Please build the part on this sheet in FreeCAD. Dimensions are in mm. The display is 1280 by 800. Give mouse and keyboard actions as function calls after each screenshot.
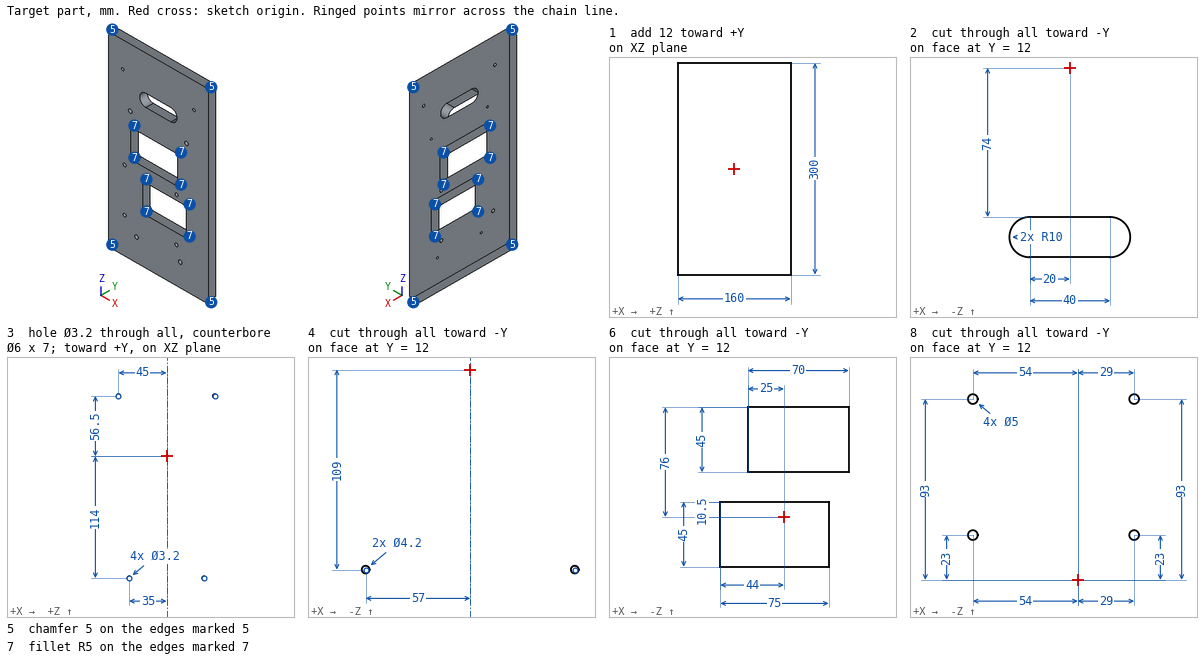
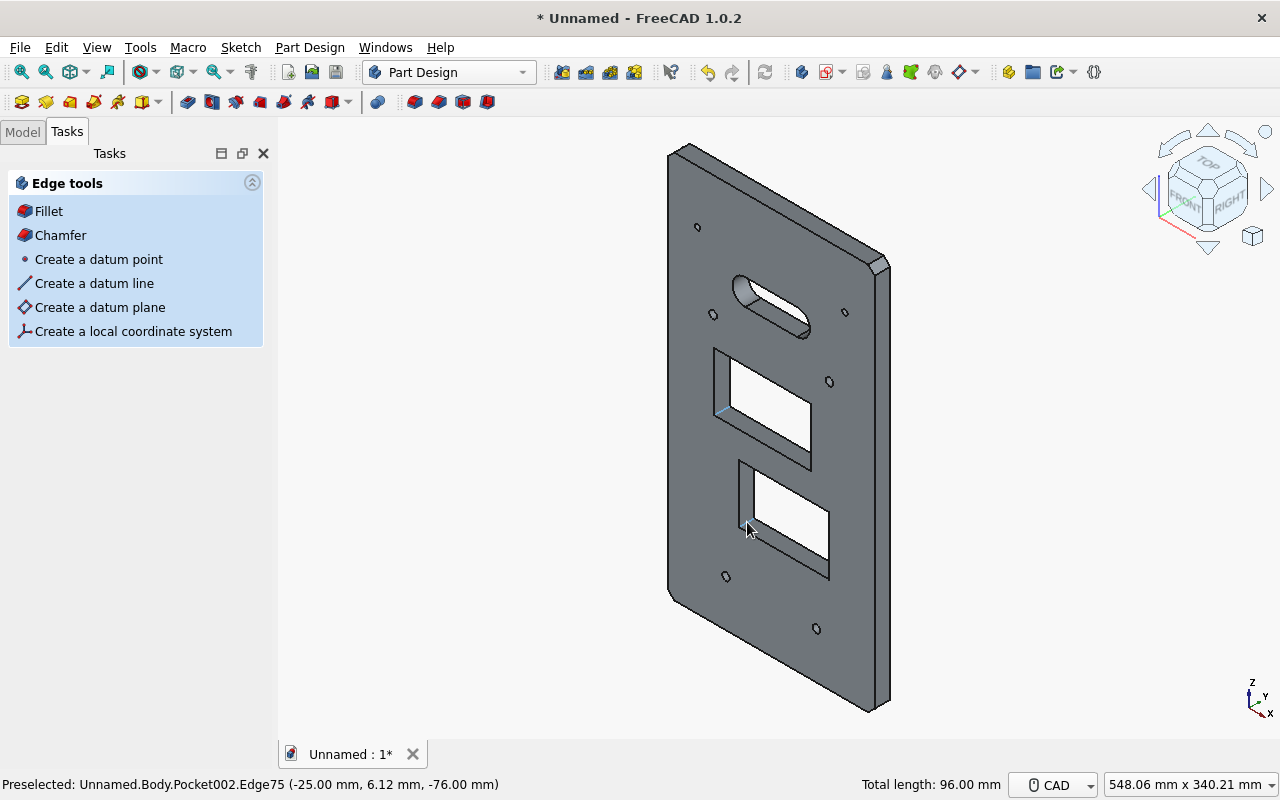
click(416, 102)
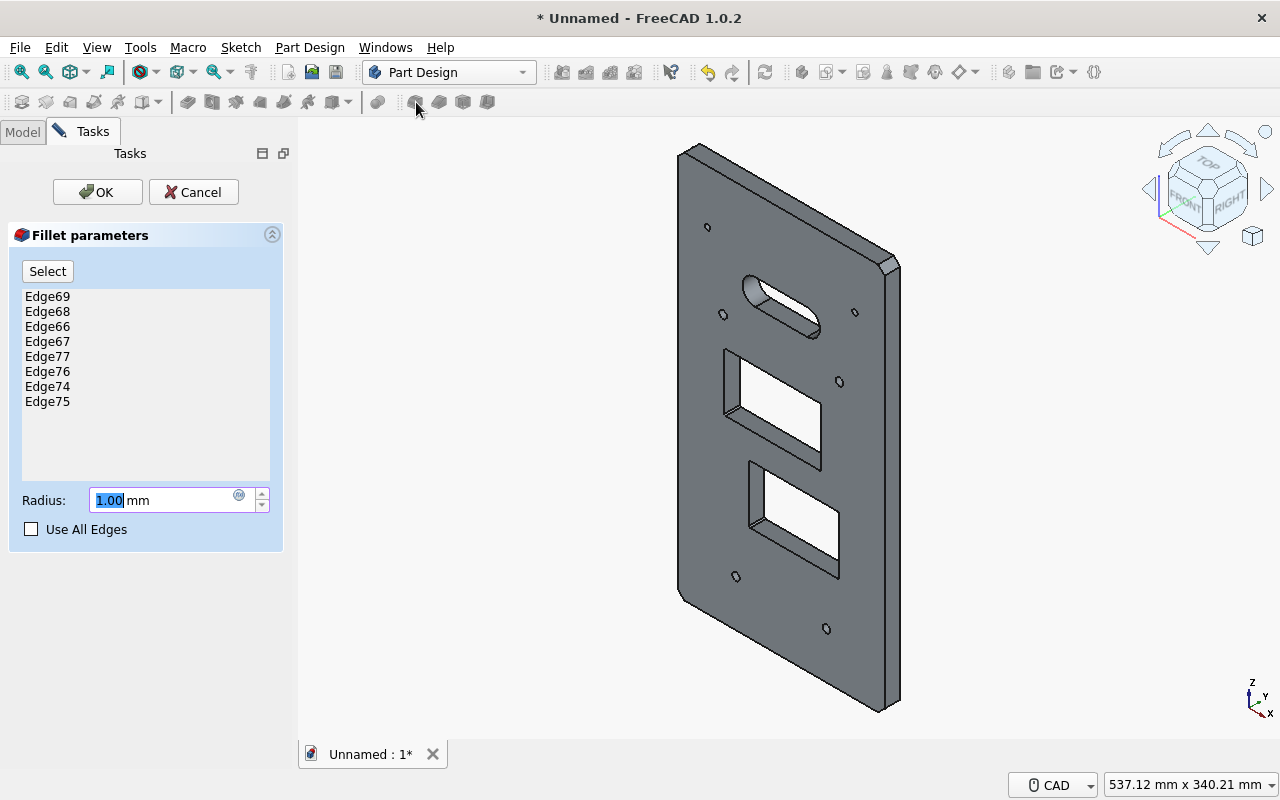
text(5)
key(Tab)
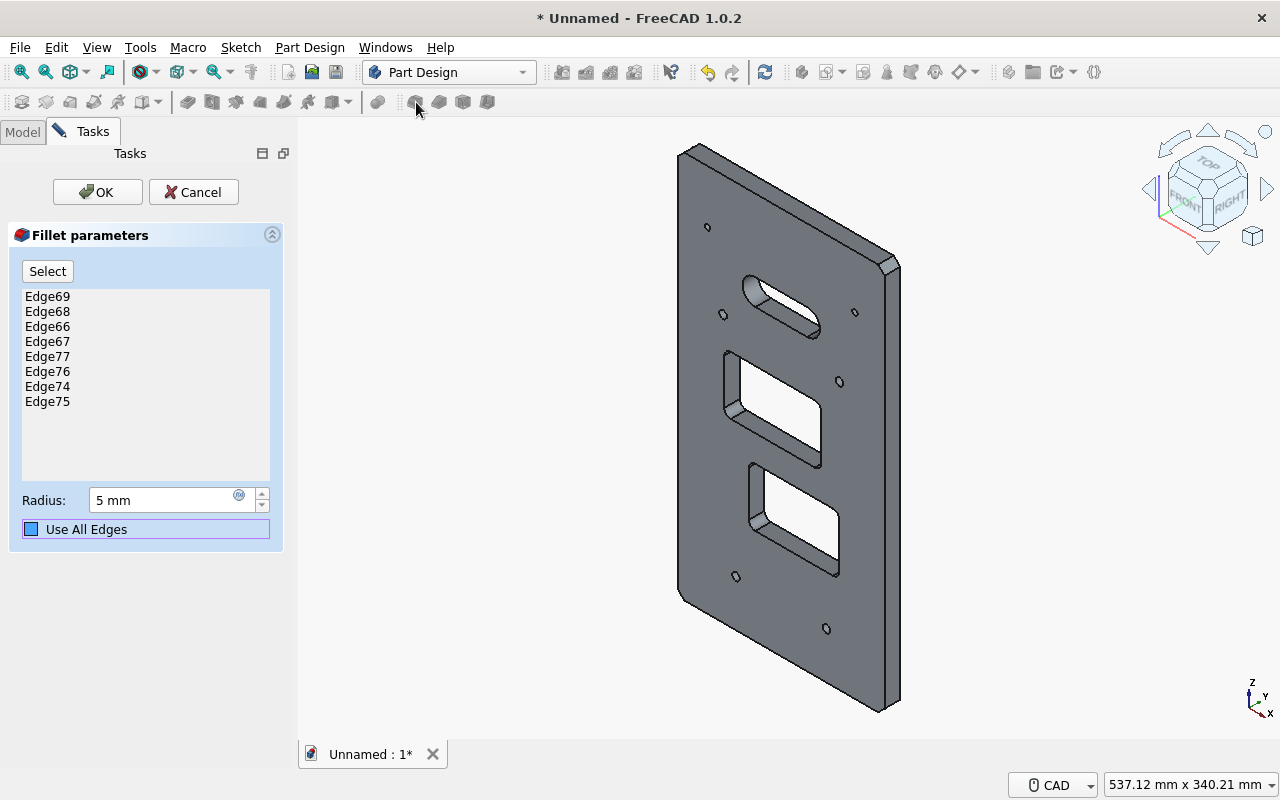
click(98, 192)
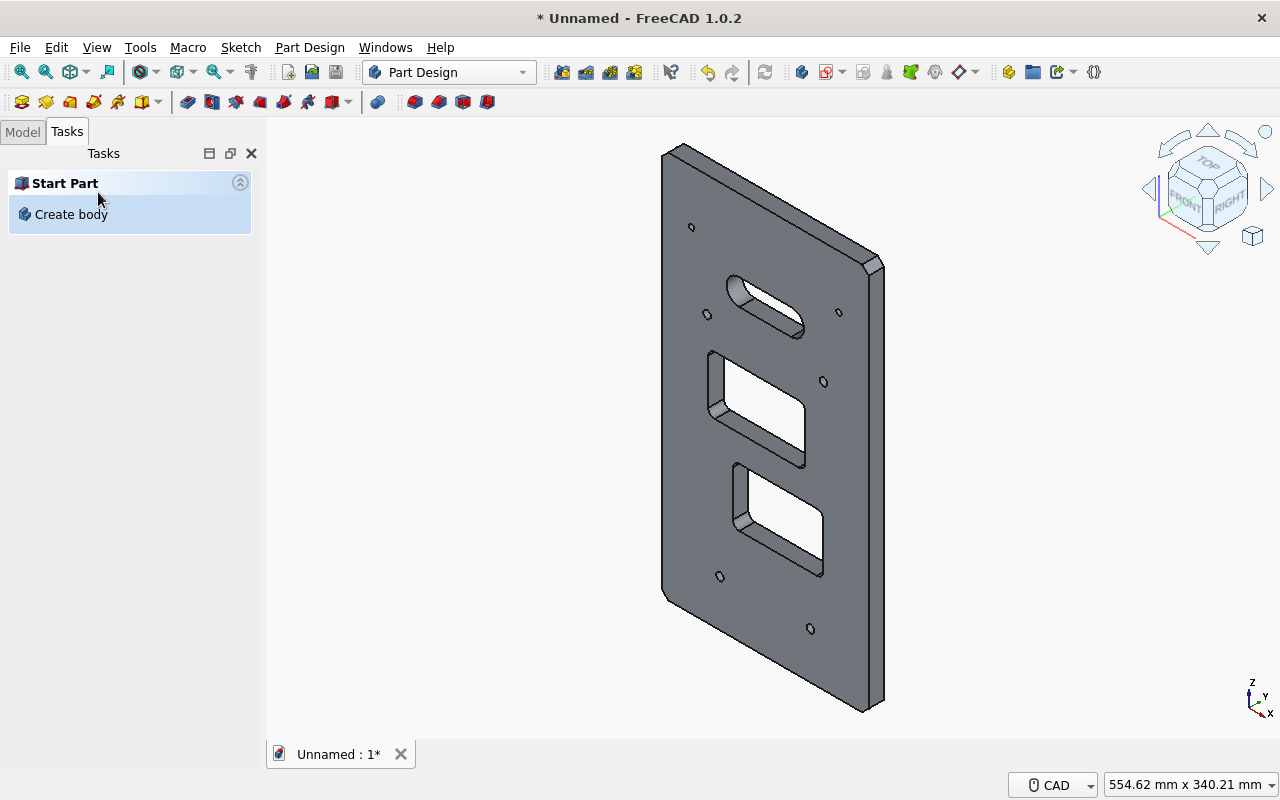
key(4)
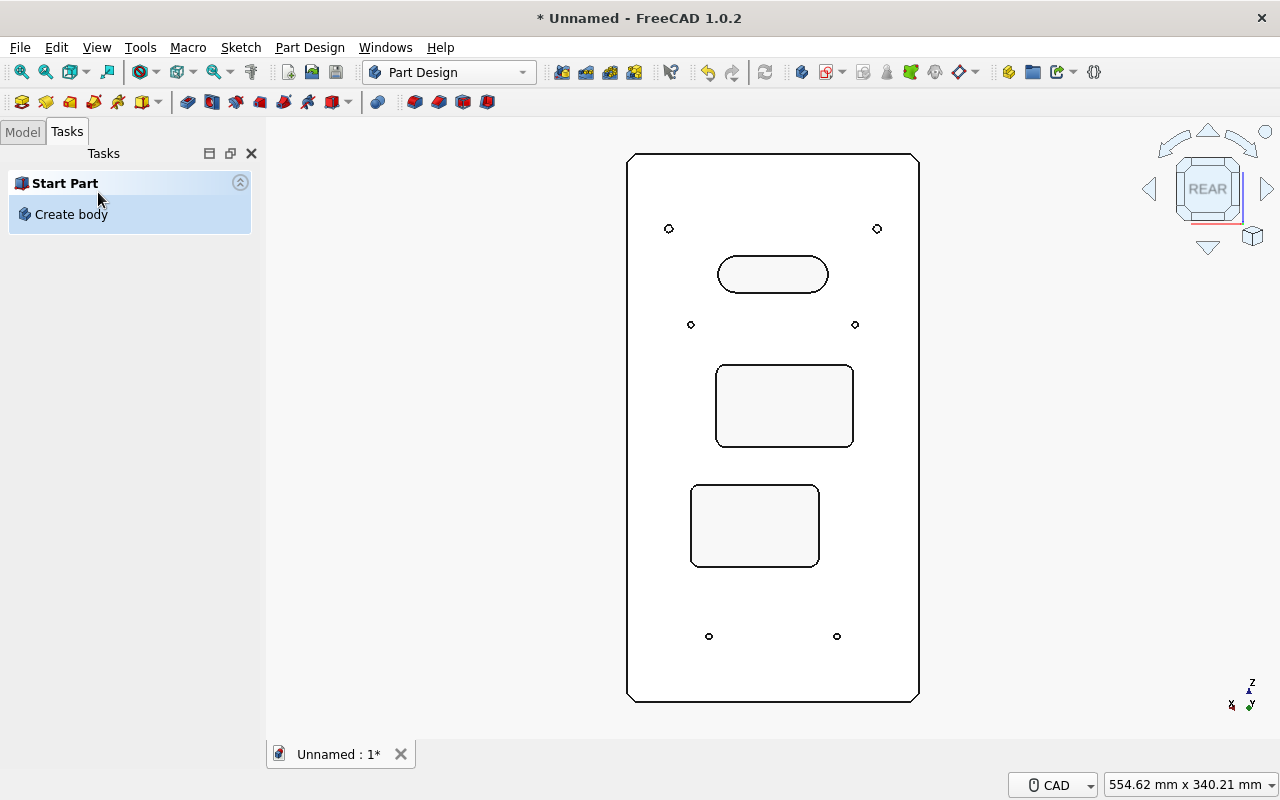
click(857, 584)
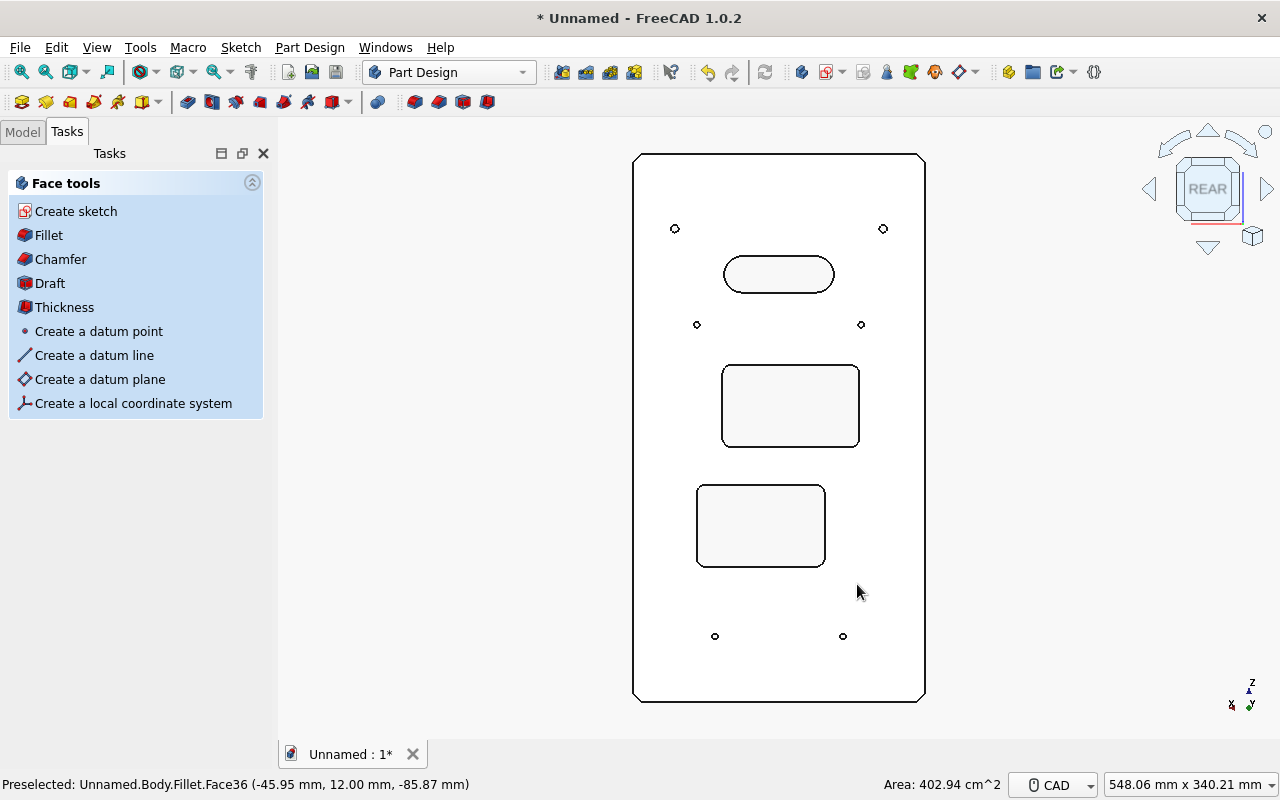
click(826, 72)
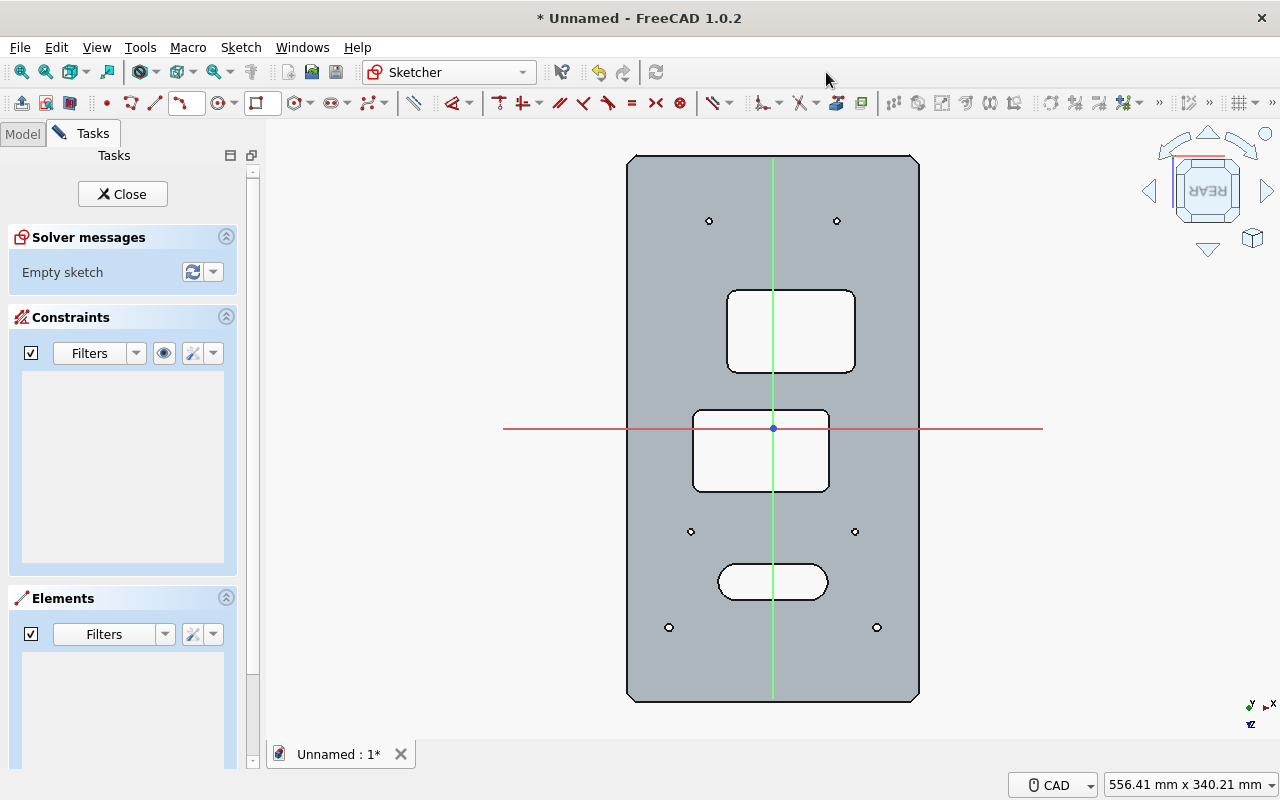
scroll(788, 271, up, 4)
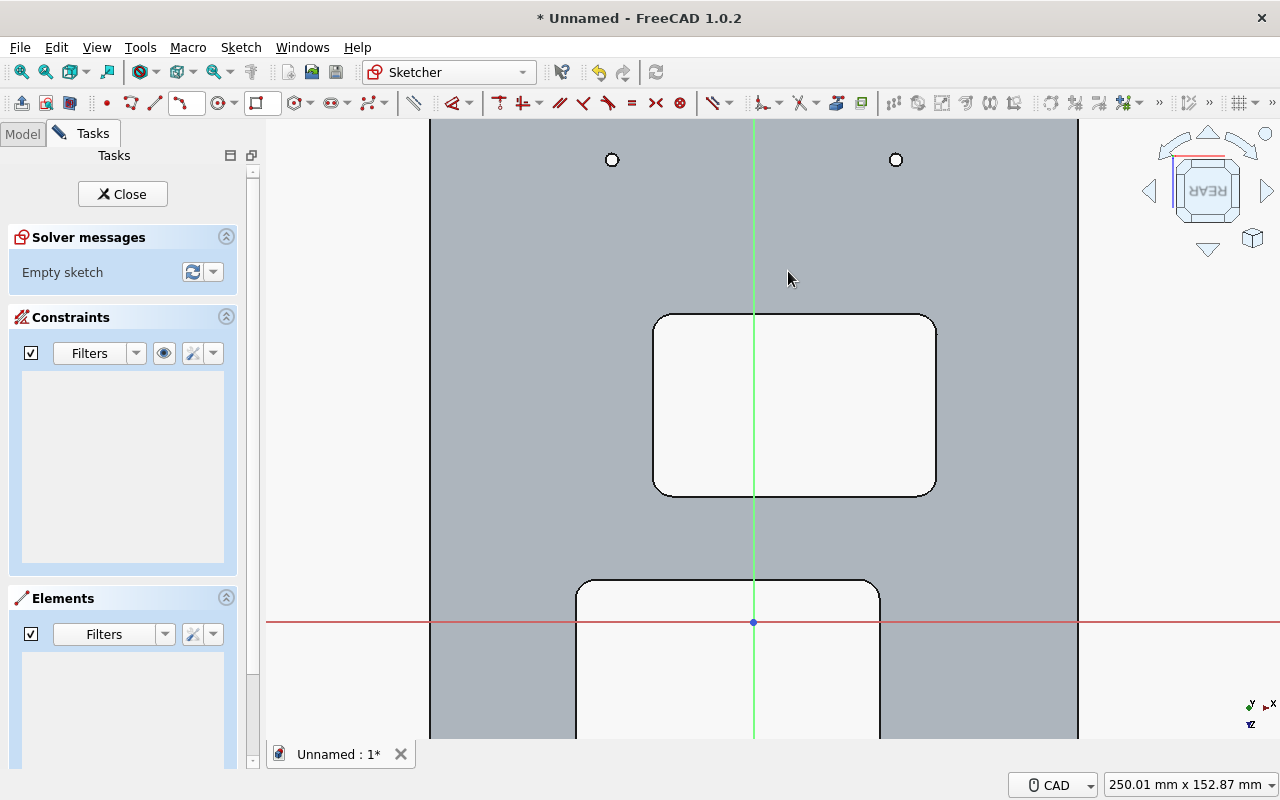
click(218, 104)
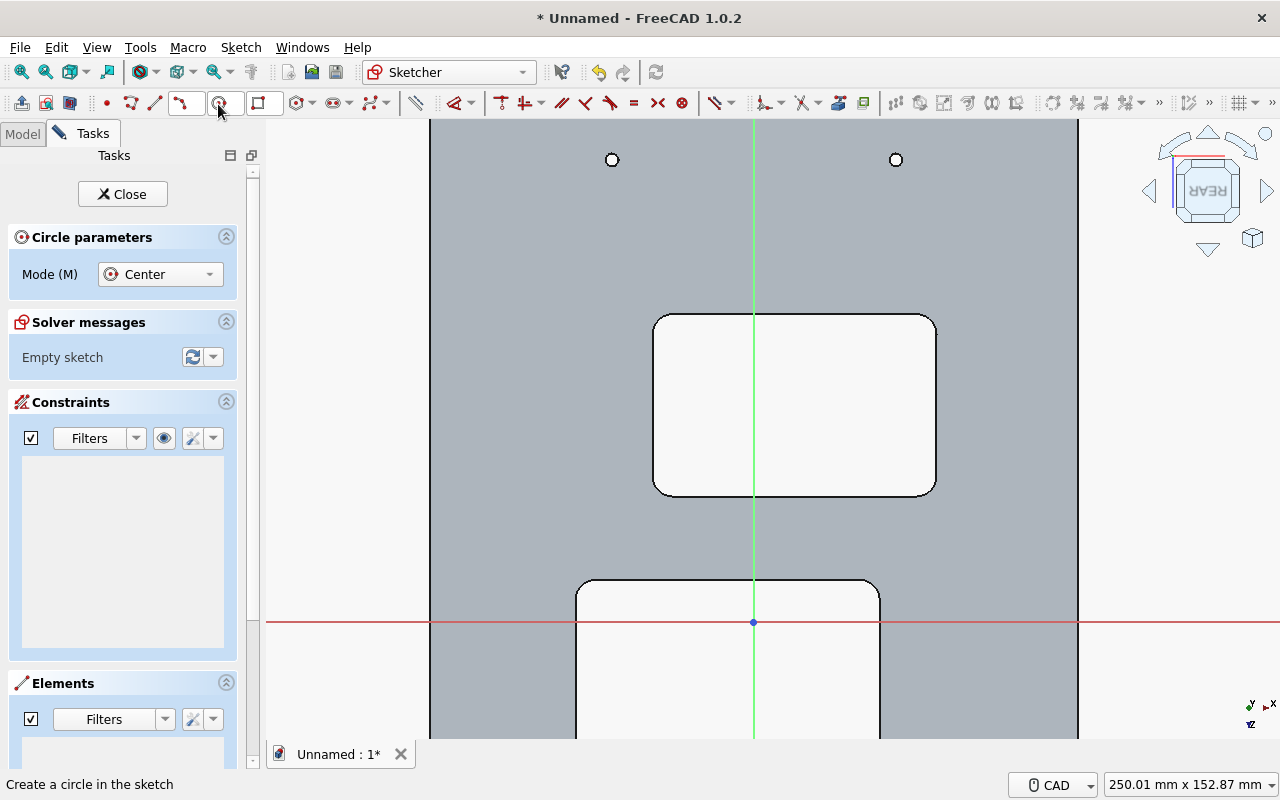
scroll(535, 245, up, 5)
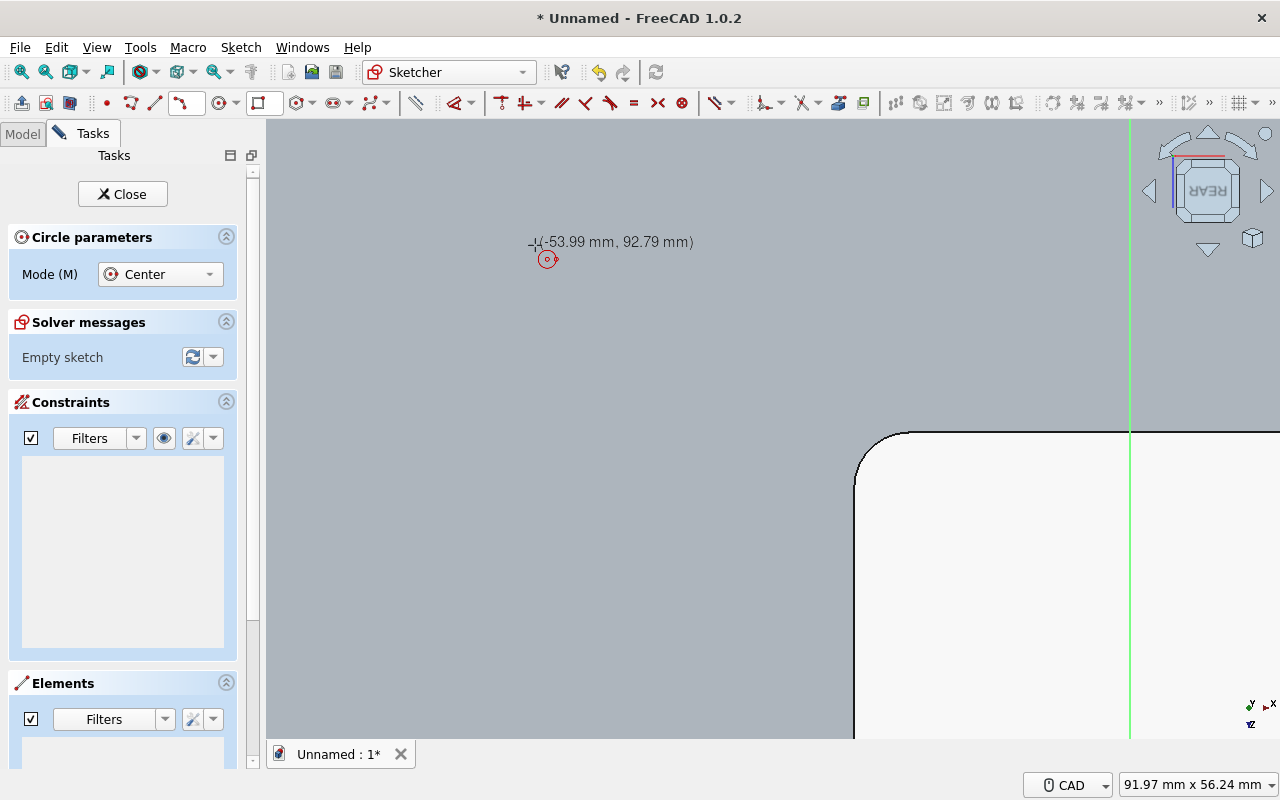
click(534, 245)
click(554, 226)